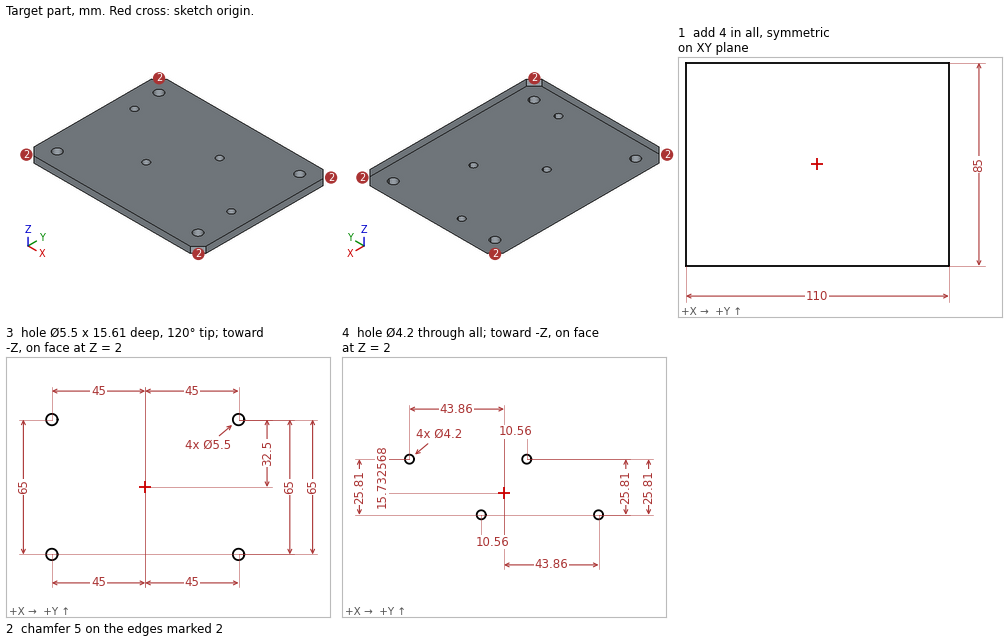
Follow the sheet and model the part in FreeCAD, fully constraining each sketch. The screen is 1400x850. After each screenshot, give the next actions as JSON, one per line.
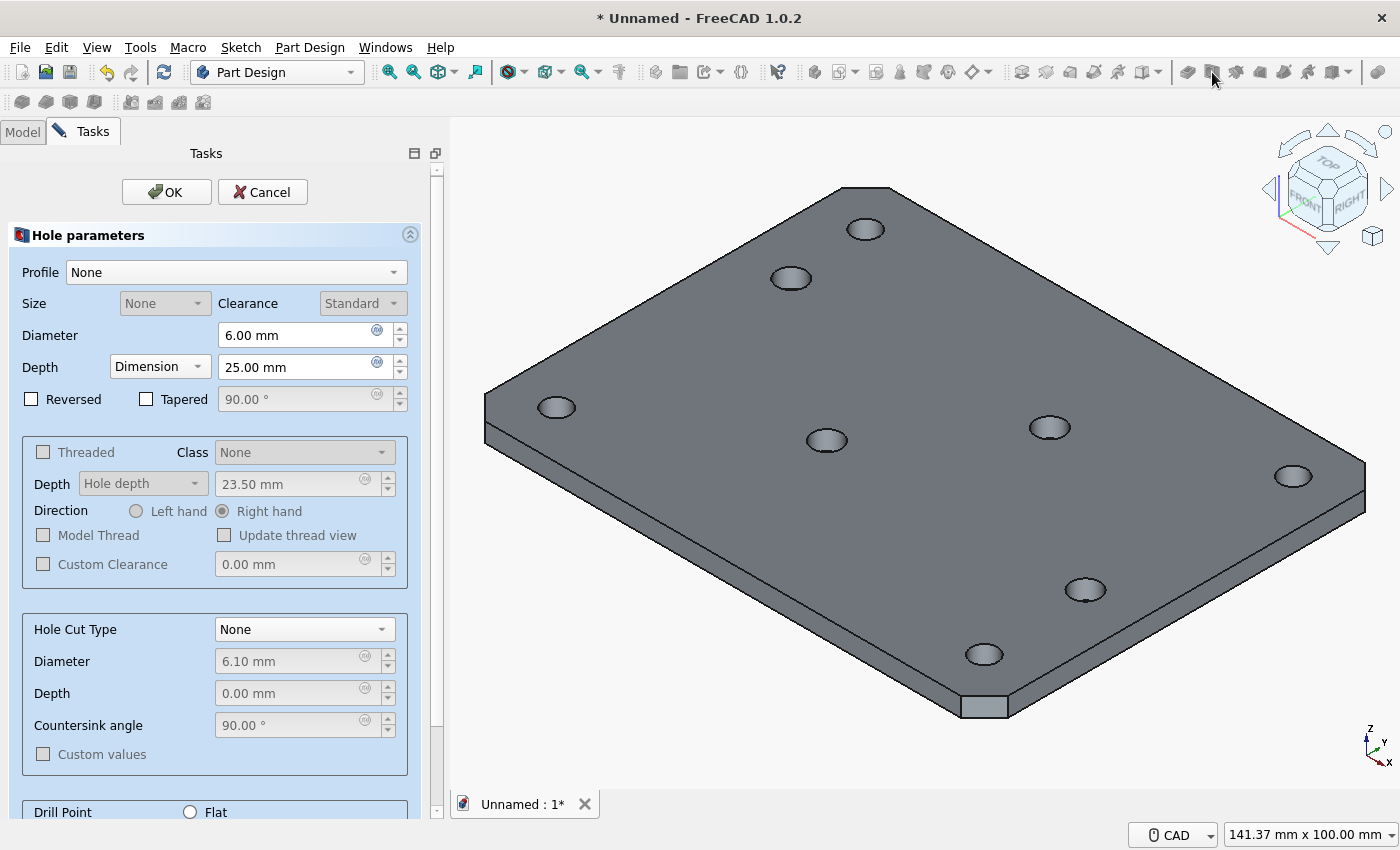
{"action": "triple_click", "coordinate": [305, 335]}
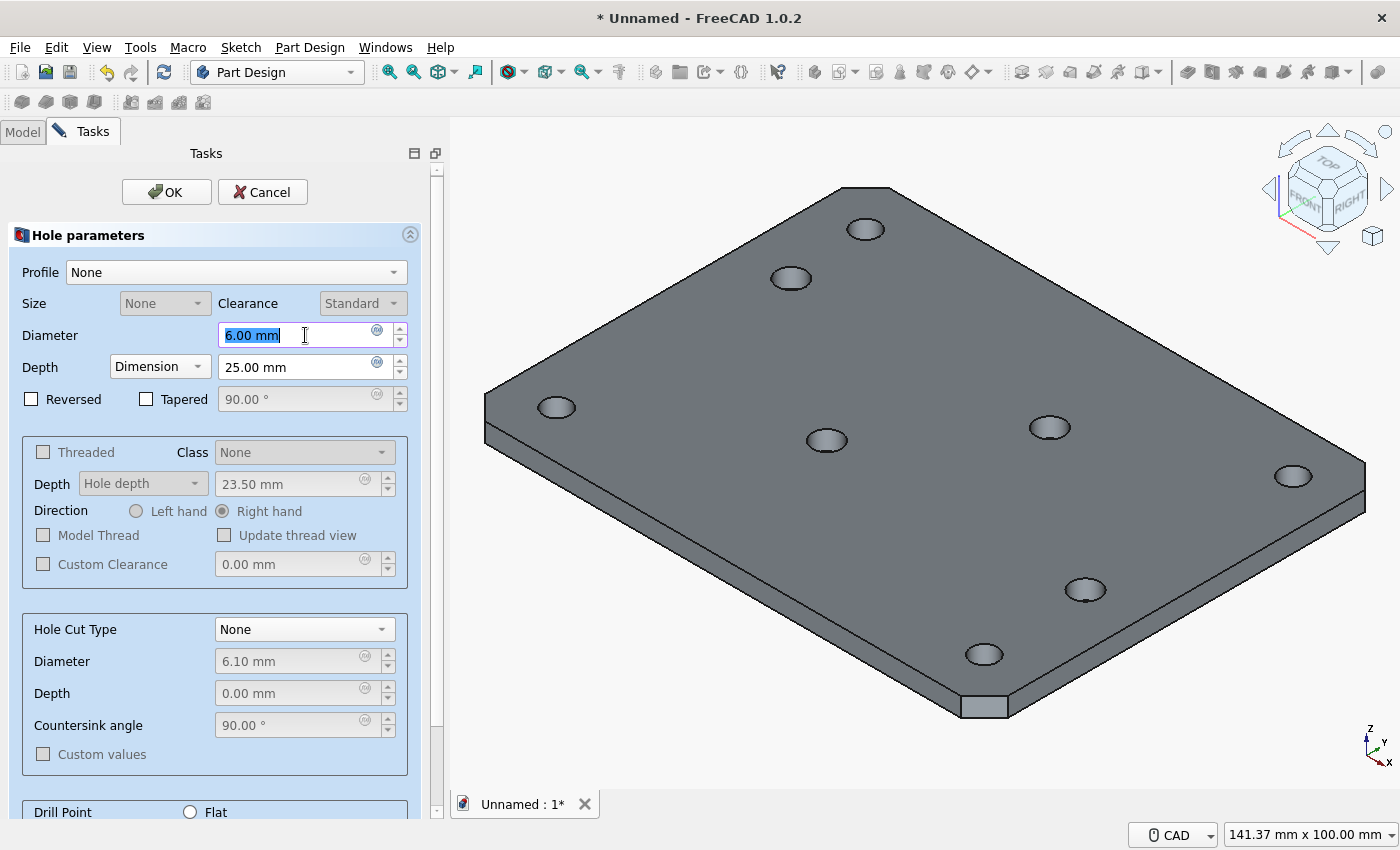
{"action": "type", "text": "4.2"}
{"action": "key", "text": "Tab"}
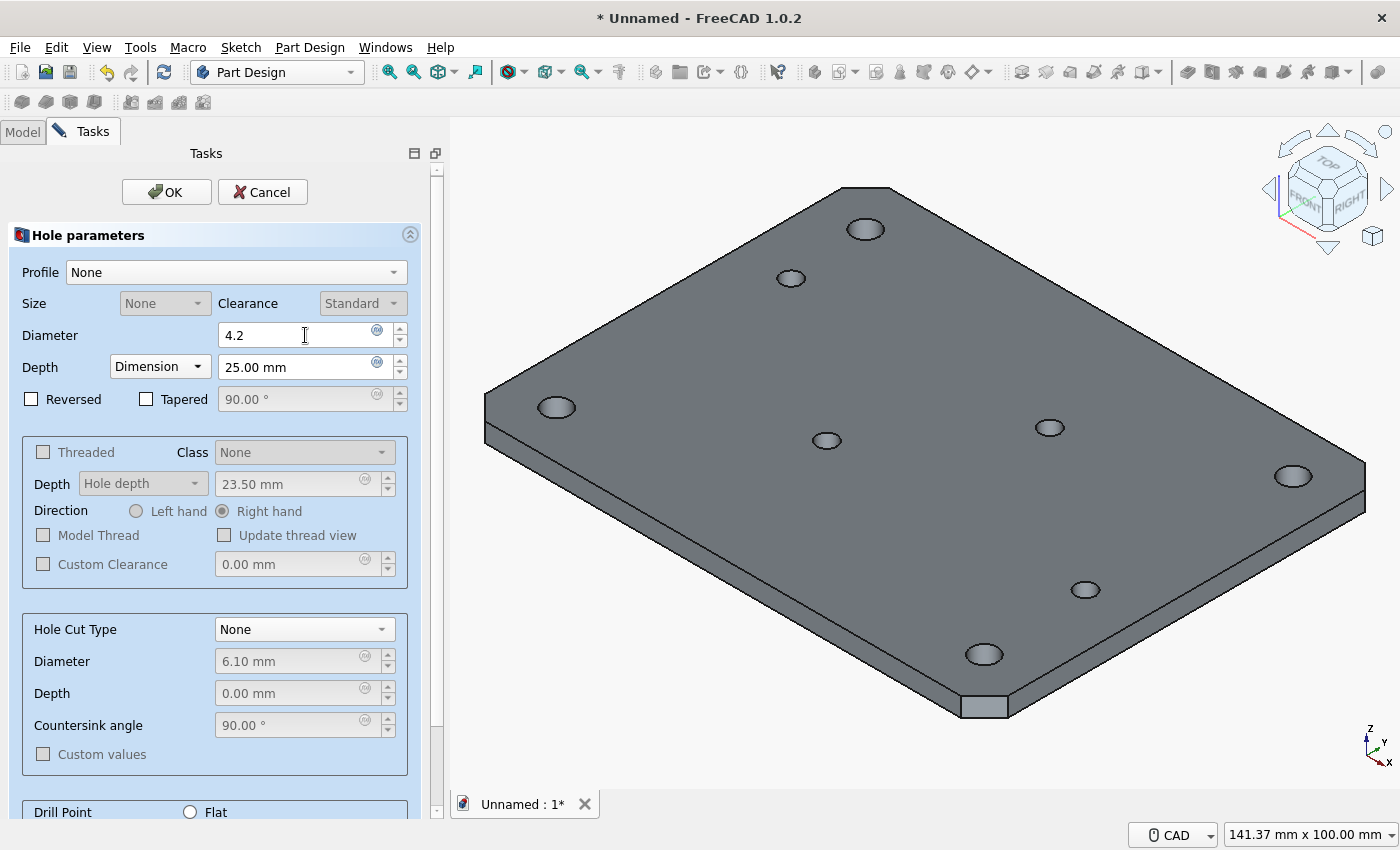
{"action": "left_click", "coordinate": [161, 366]}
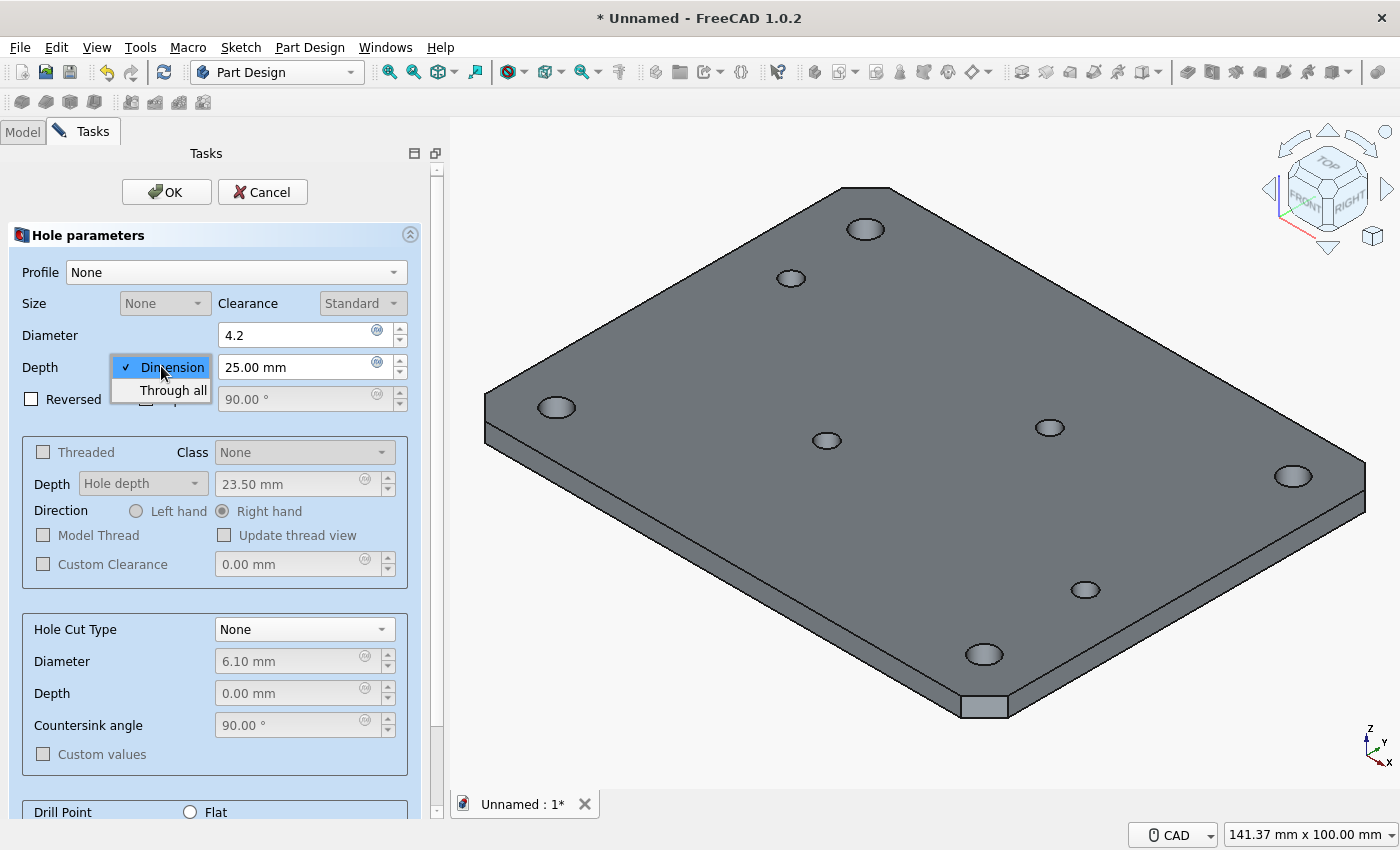
{"action": "left_click", "coordinate": [160, 390]}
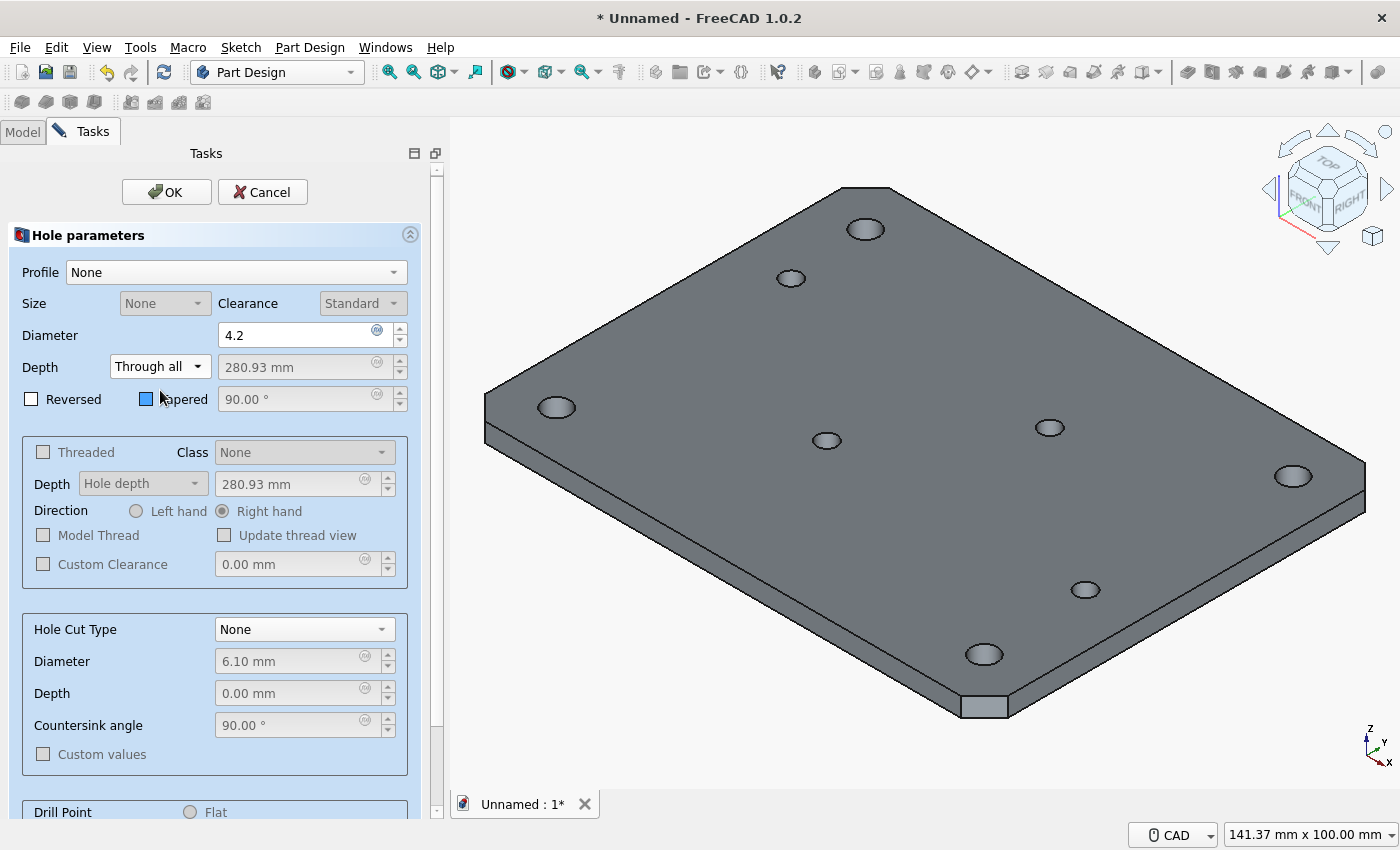
{"action": "left_click", "coordinate": [167, 192]}